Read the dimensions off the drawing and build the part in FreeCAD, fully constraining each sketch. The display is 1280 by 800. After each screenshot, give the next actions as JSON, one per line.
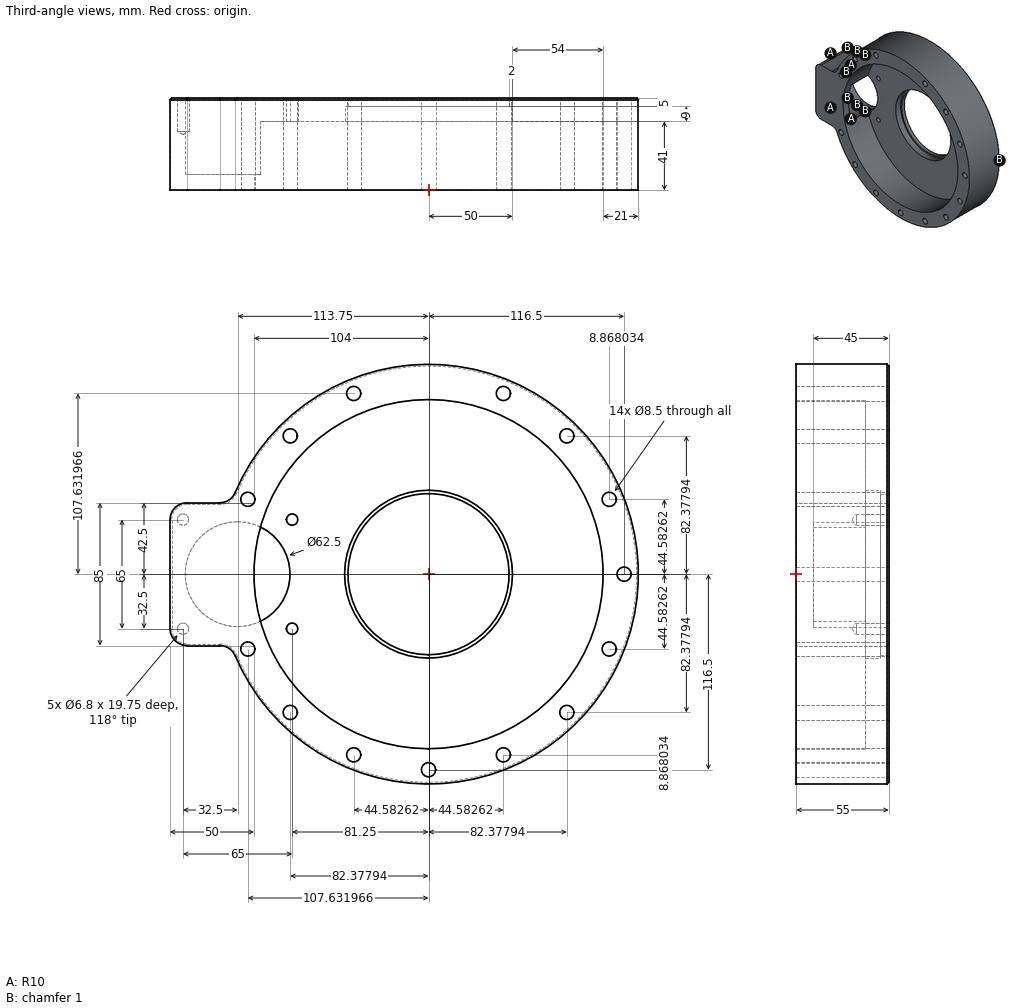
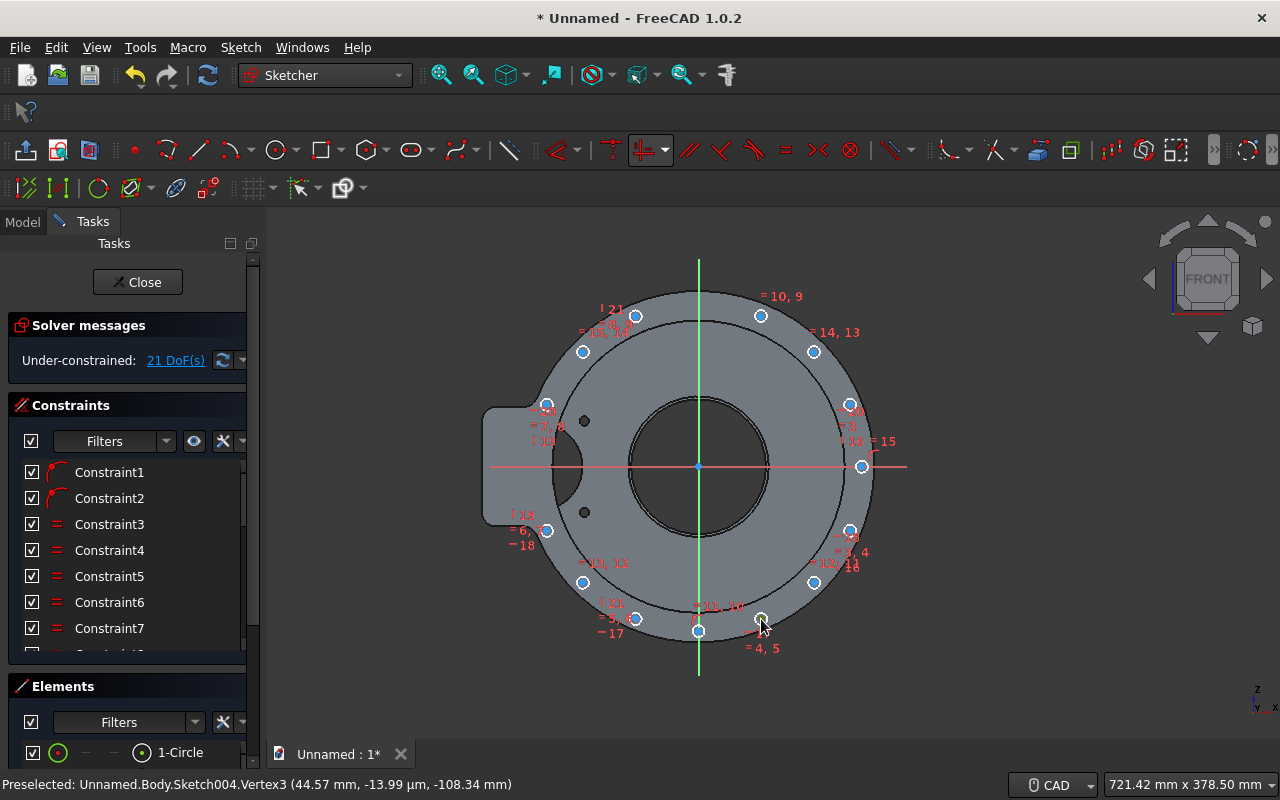
{"action": "left_click", "coordinate": [761, 316]}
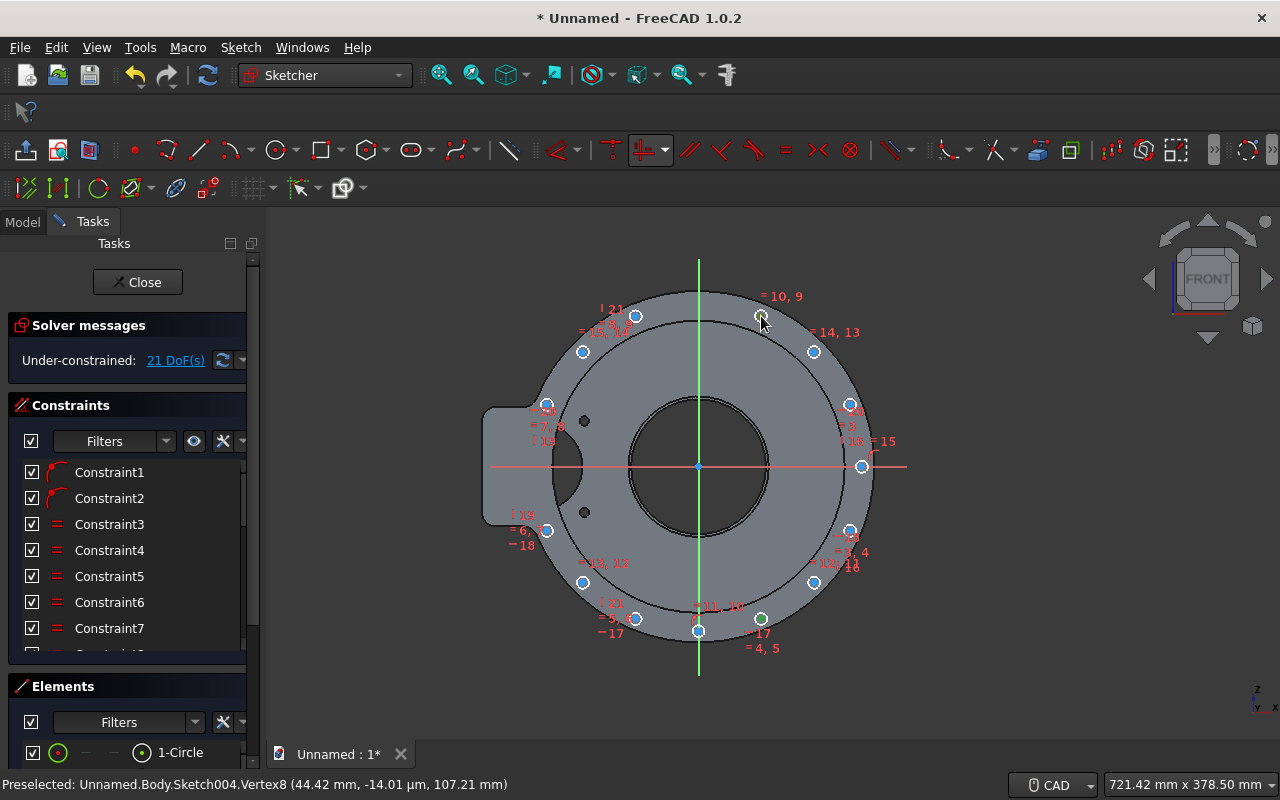
{"action": "key", "text": "v"}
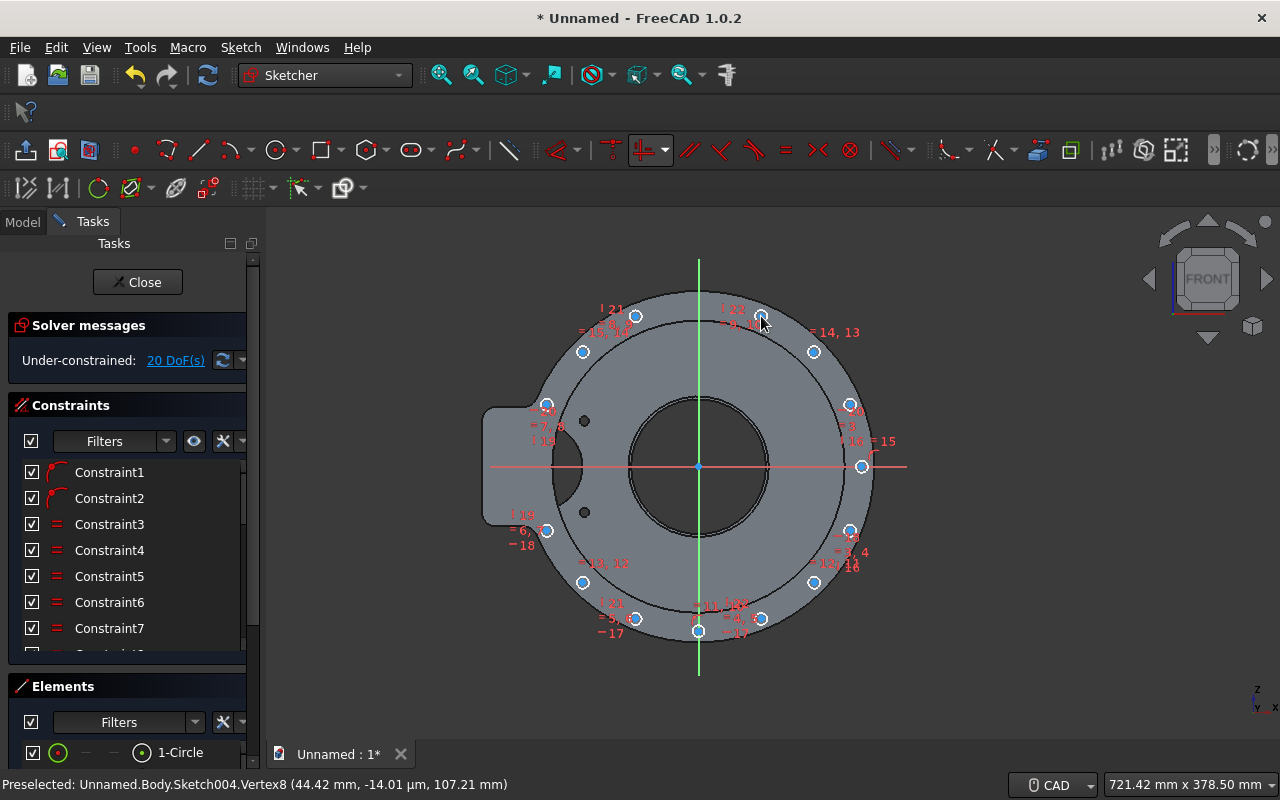
{"action": "left_click", "coordinate": [636, 316]}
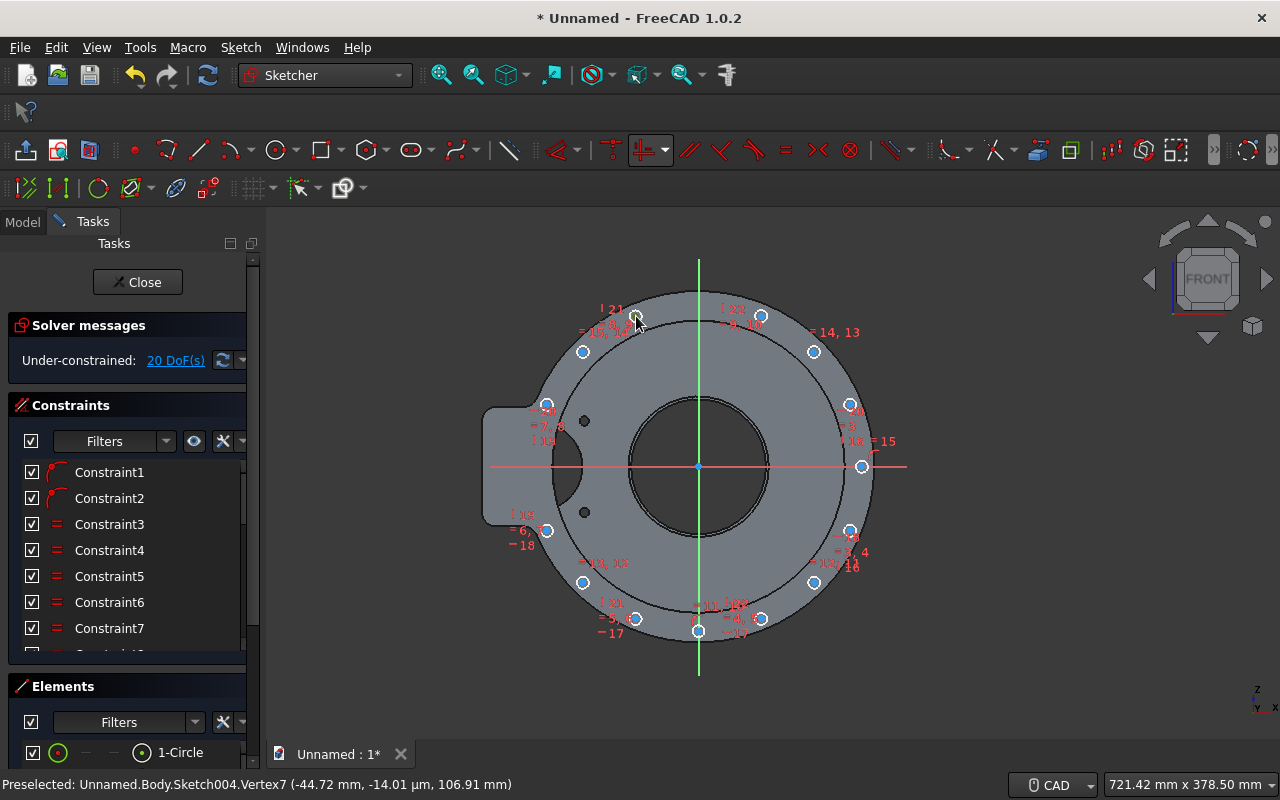
{"action": "left_click", "coordinate": [763, 318]}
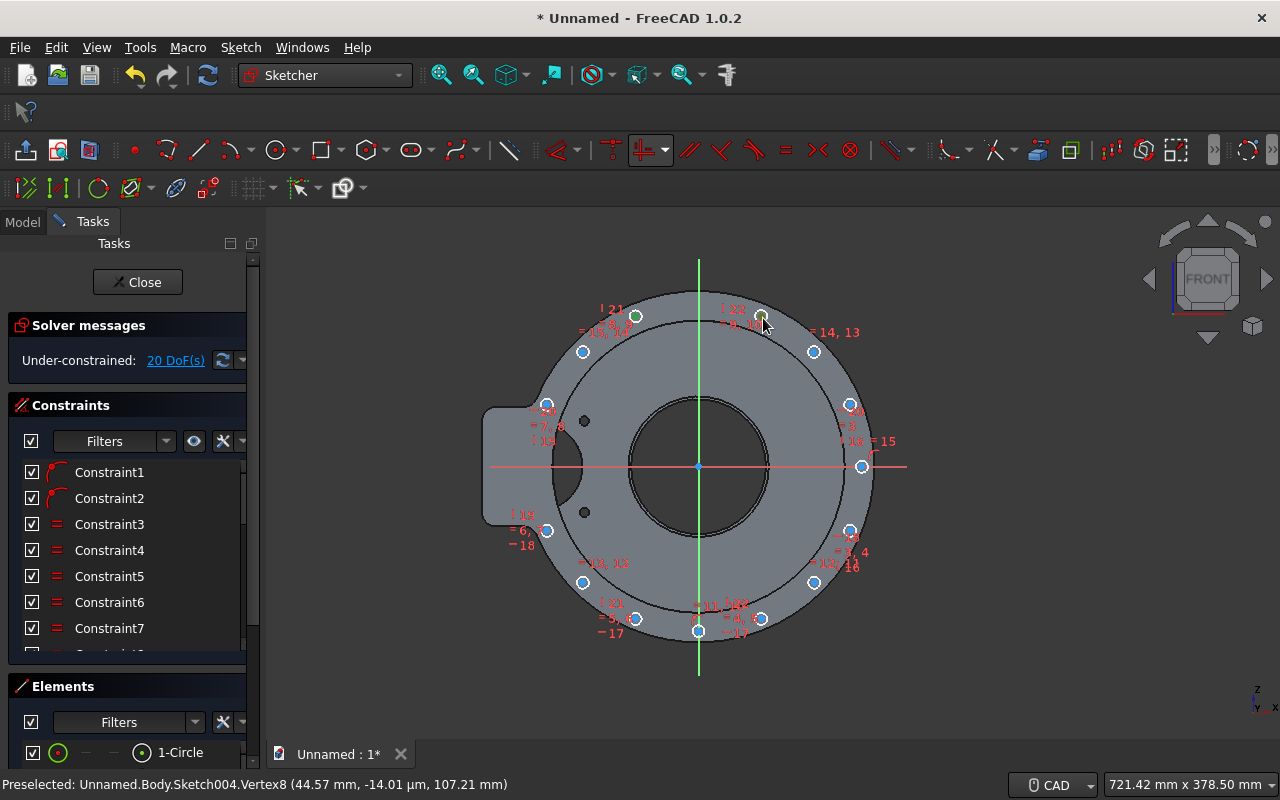
{"action": "key", "text": "h"}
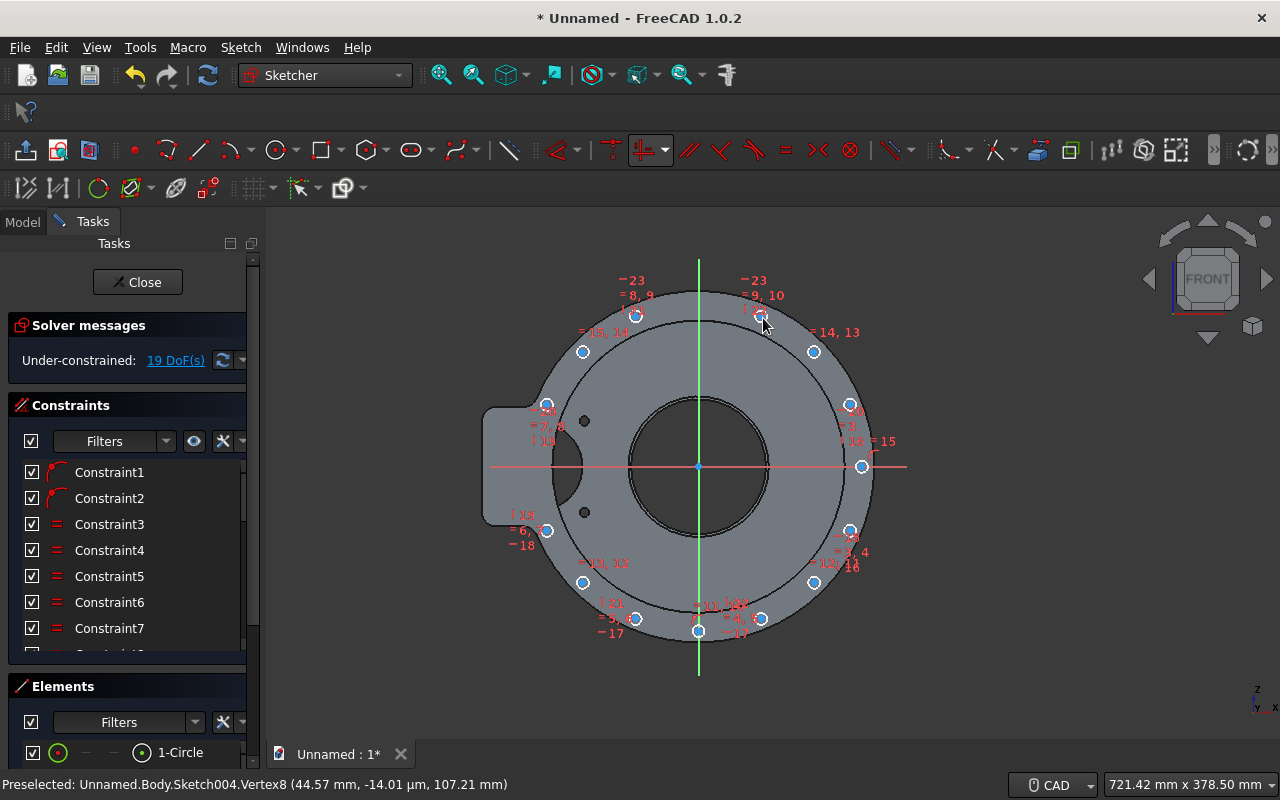
{"action": "left_click", "coordinate": [814, 583]}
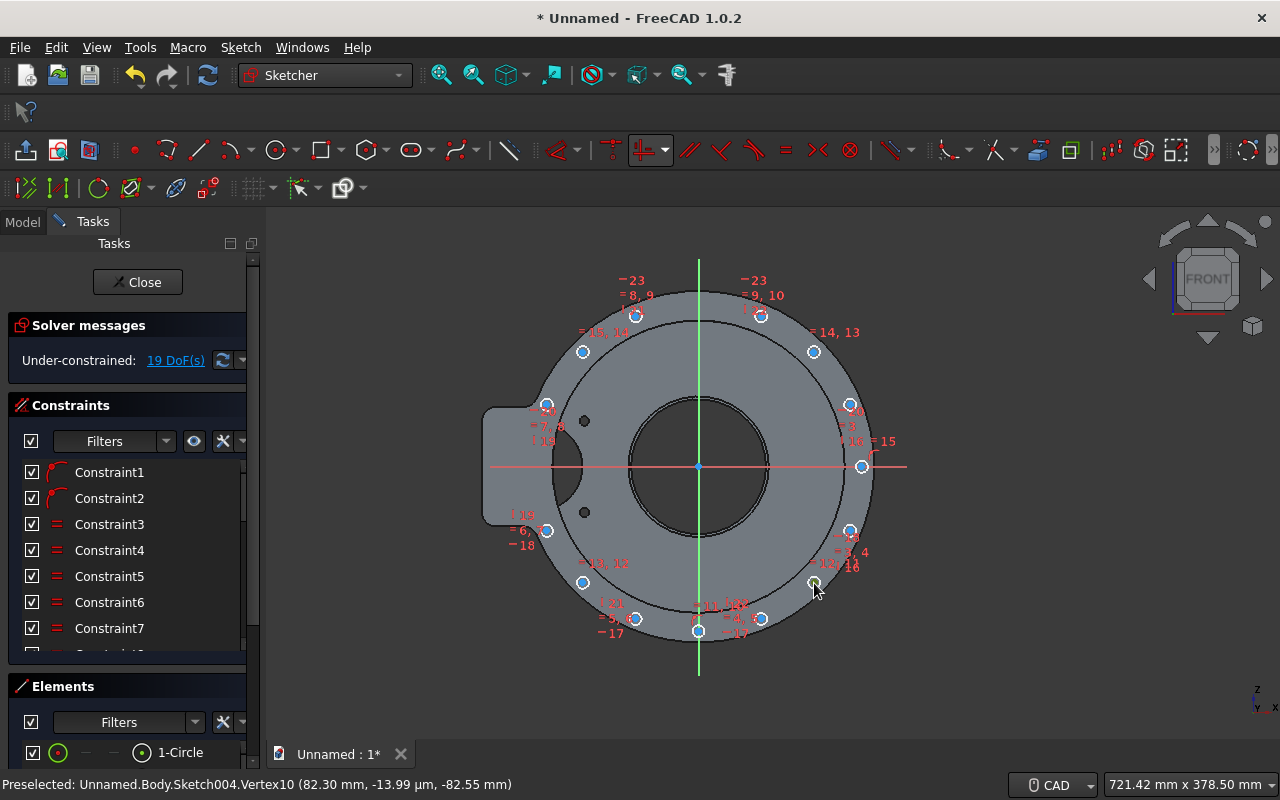
{"action": "left_click", "coordinate": [583, 583]}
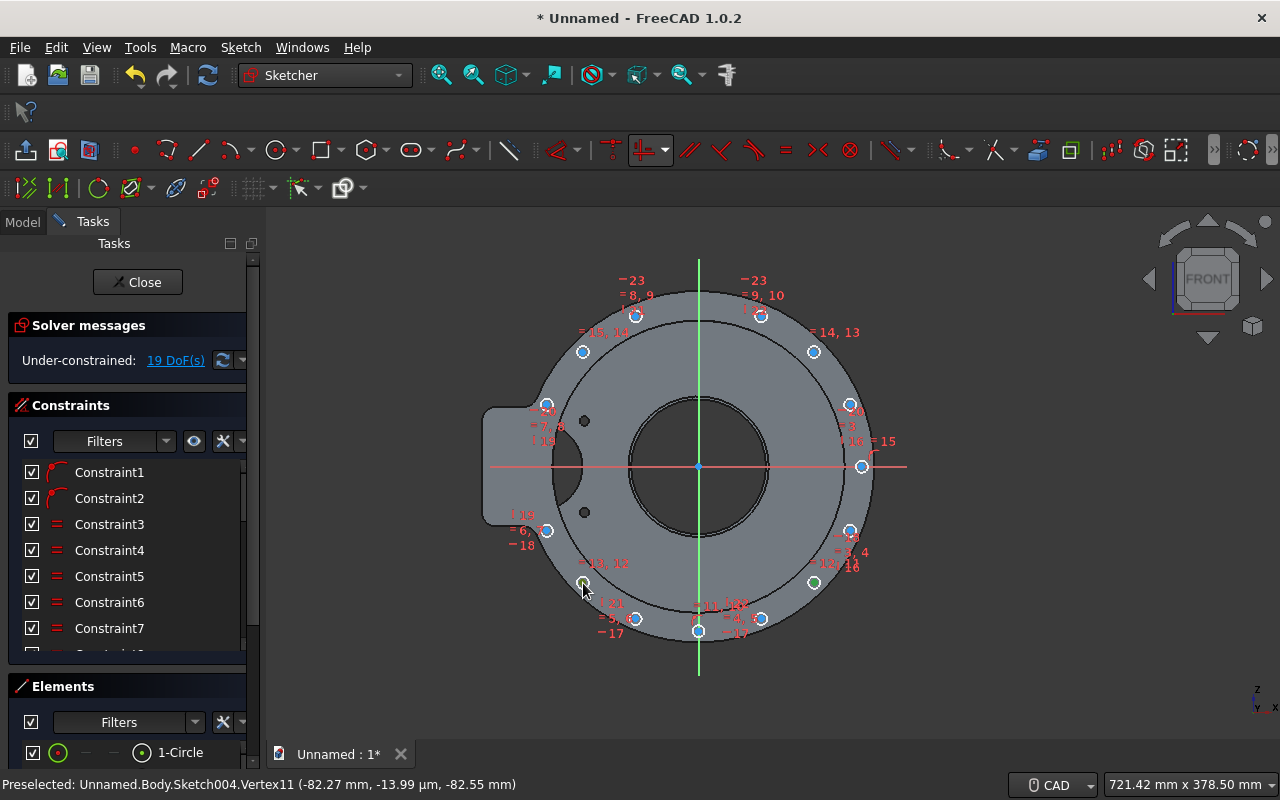
{"action": "left_click", "coordinate": [668, 150]}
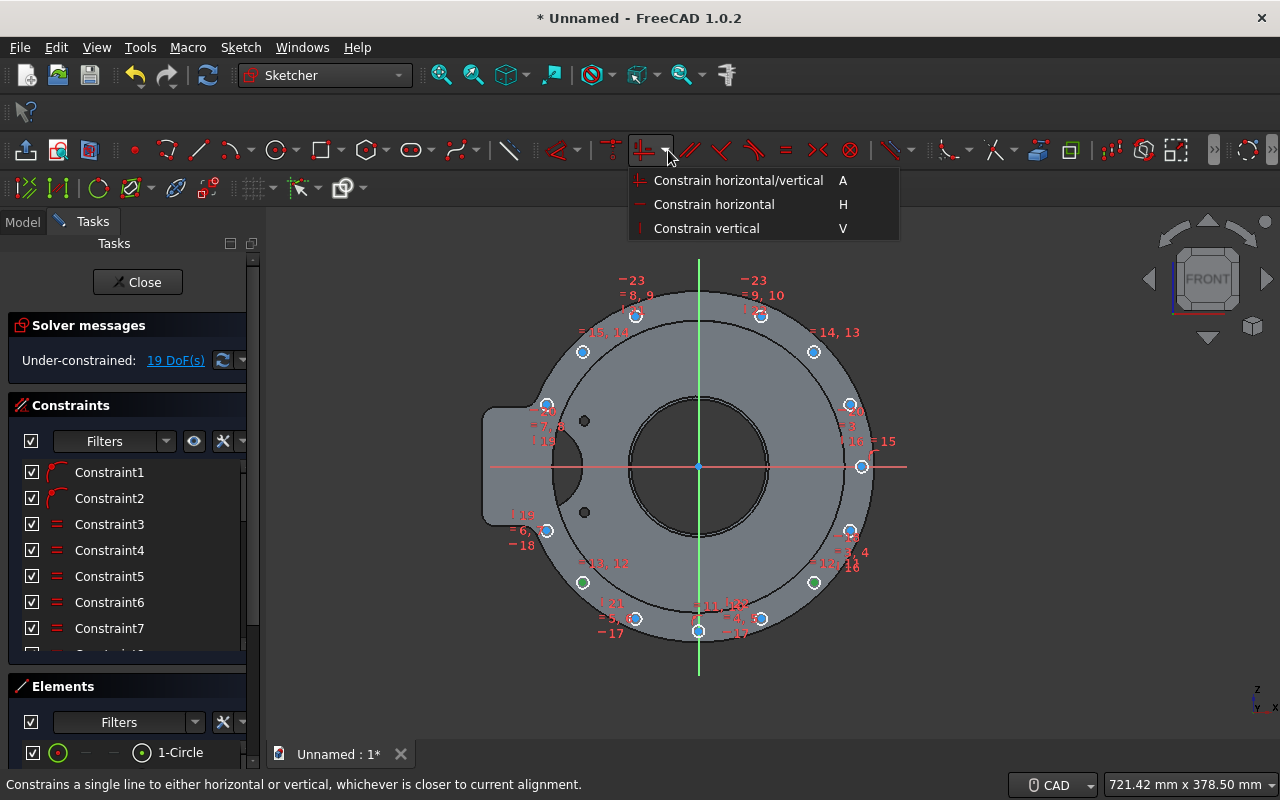
{"action": "left_click", "coordinate": [764, 204]}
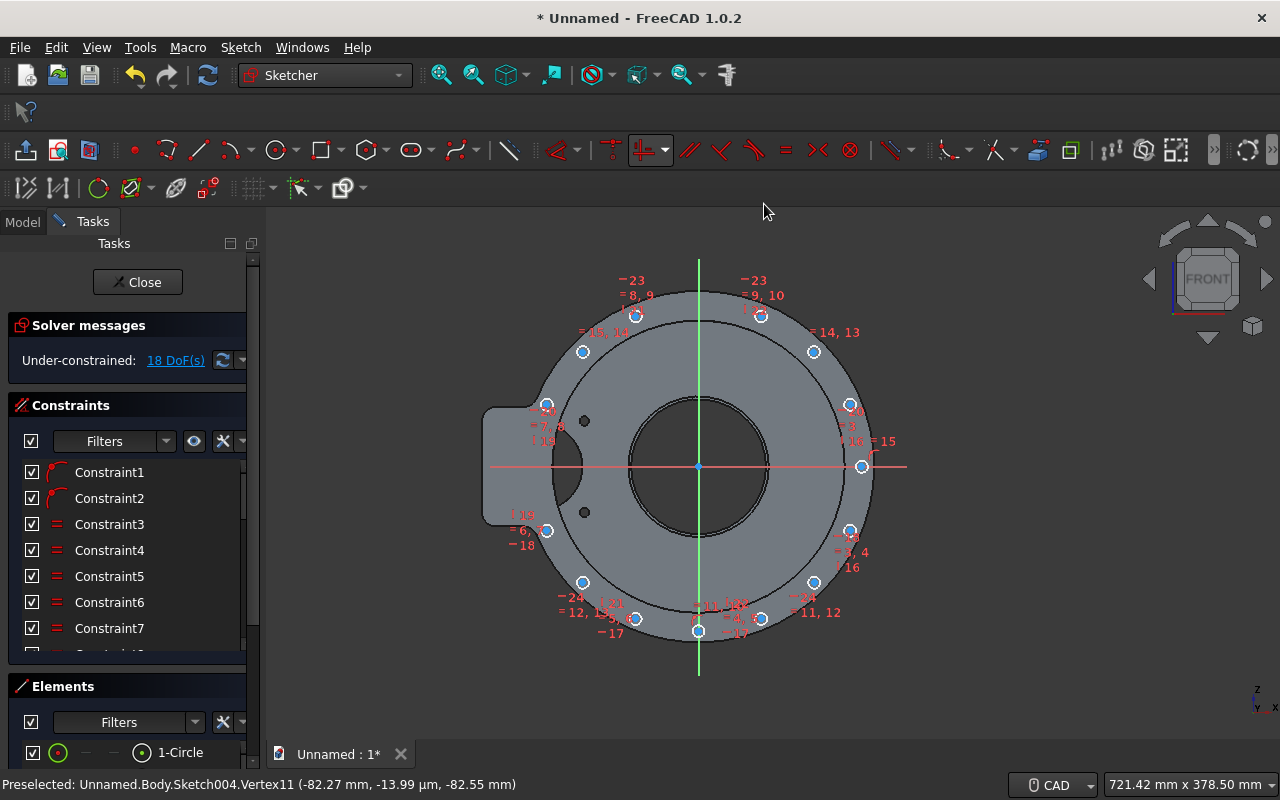
{"action": "left_click", "coordinate": [814, 583]}